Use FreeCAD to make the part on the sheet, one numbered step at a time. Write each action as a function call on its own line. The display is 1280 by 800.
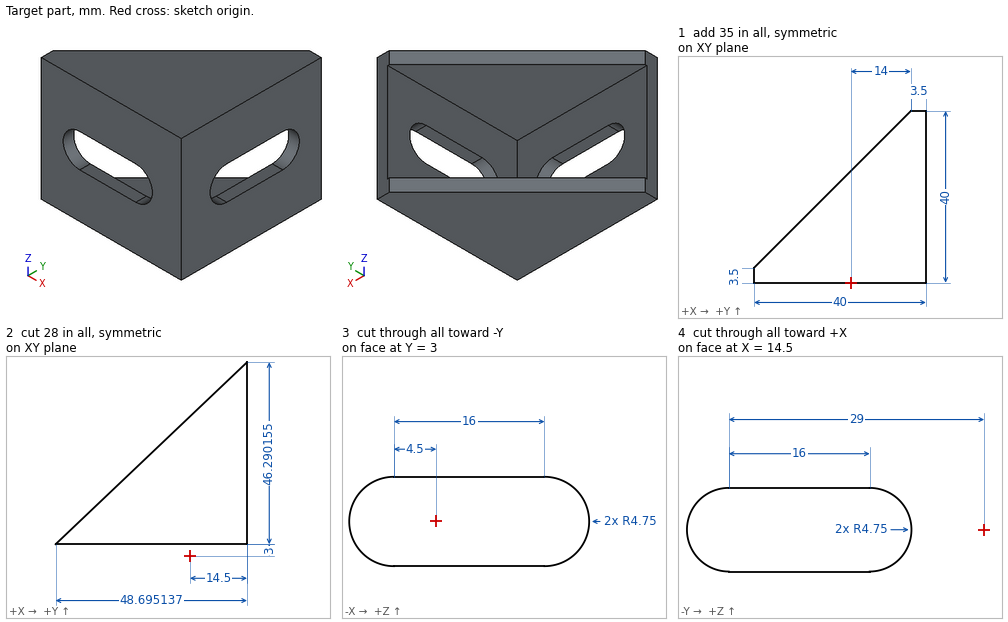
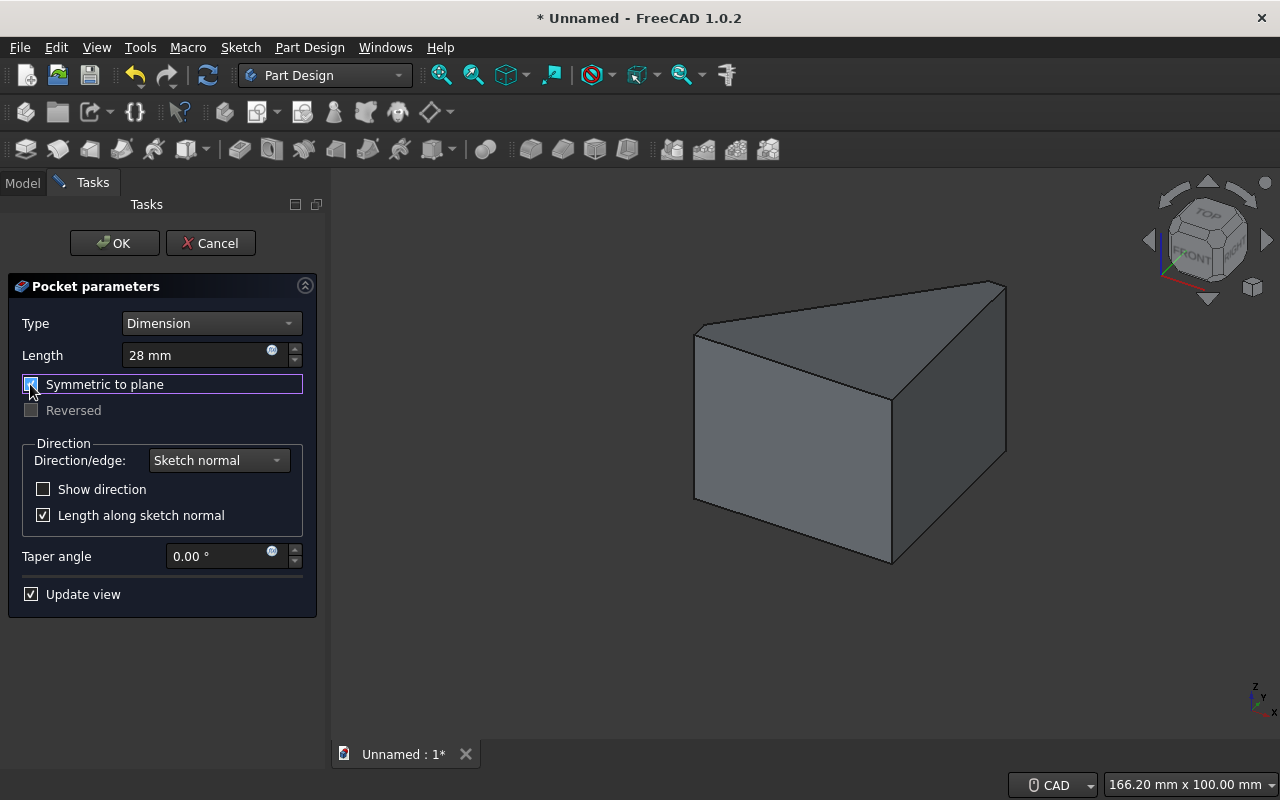
click(115, 243)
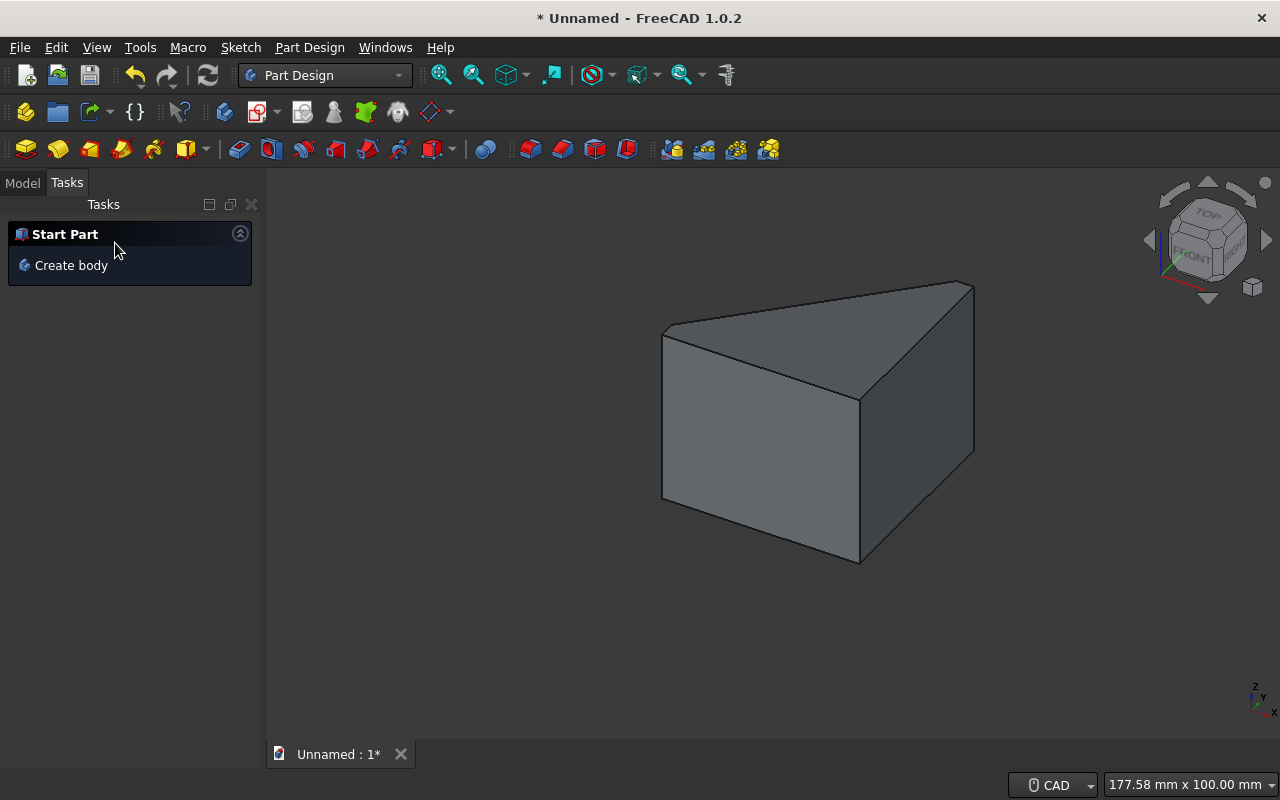
key(4)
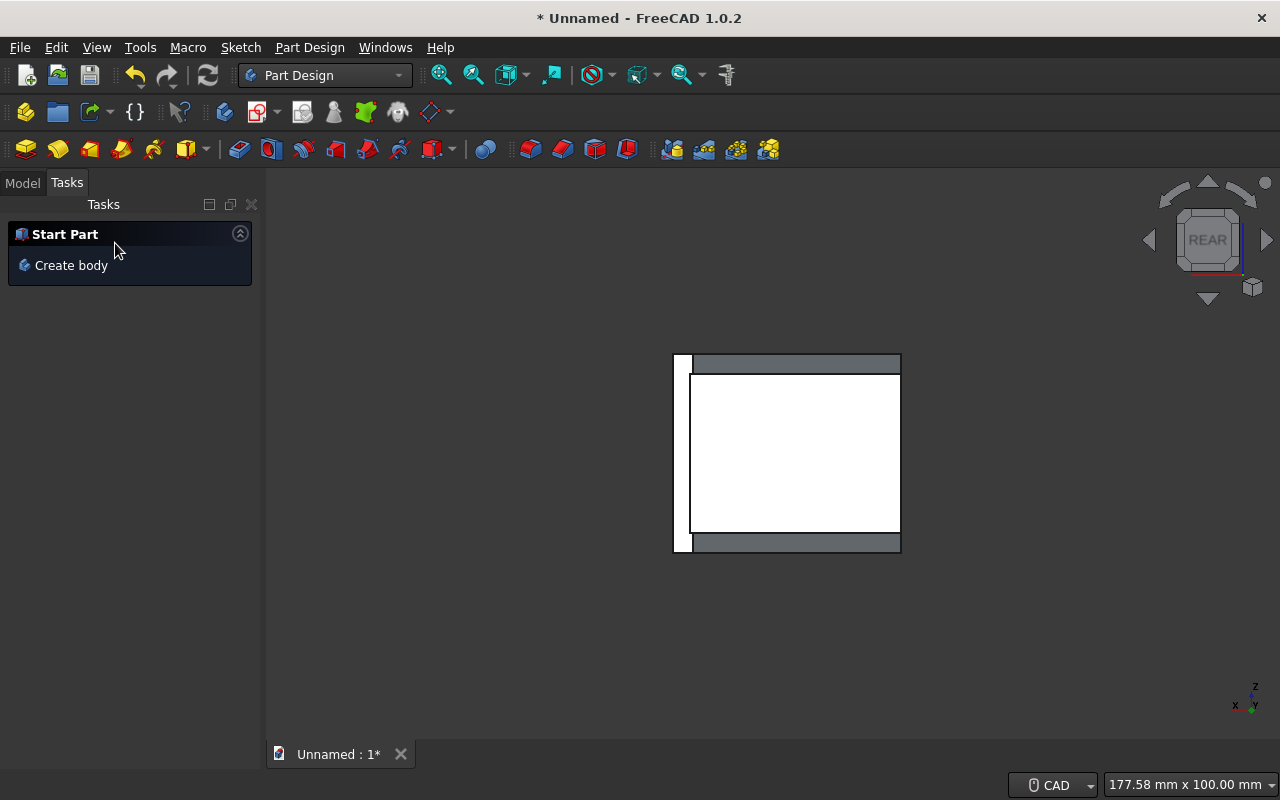
click(442, 76)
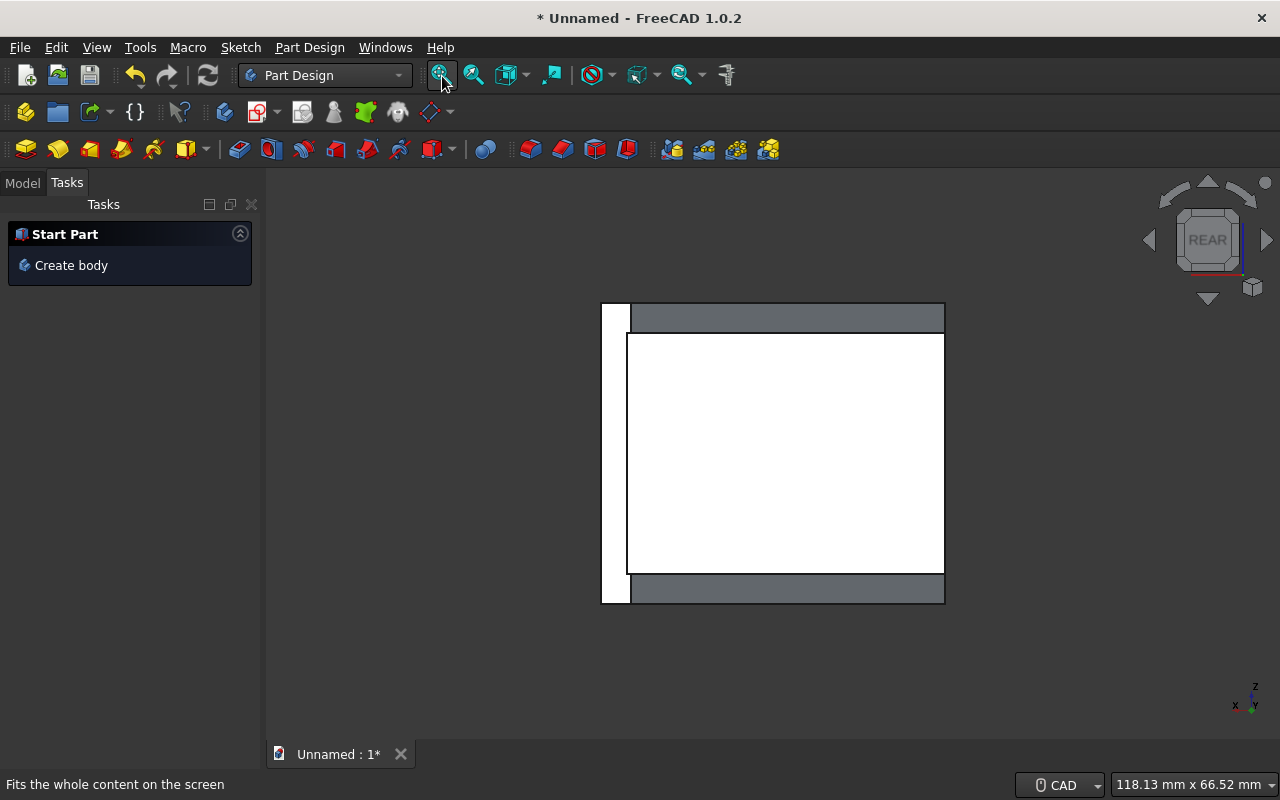
click(786, 453)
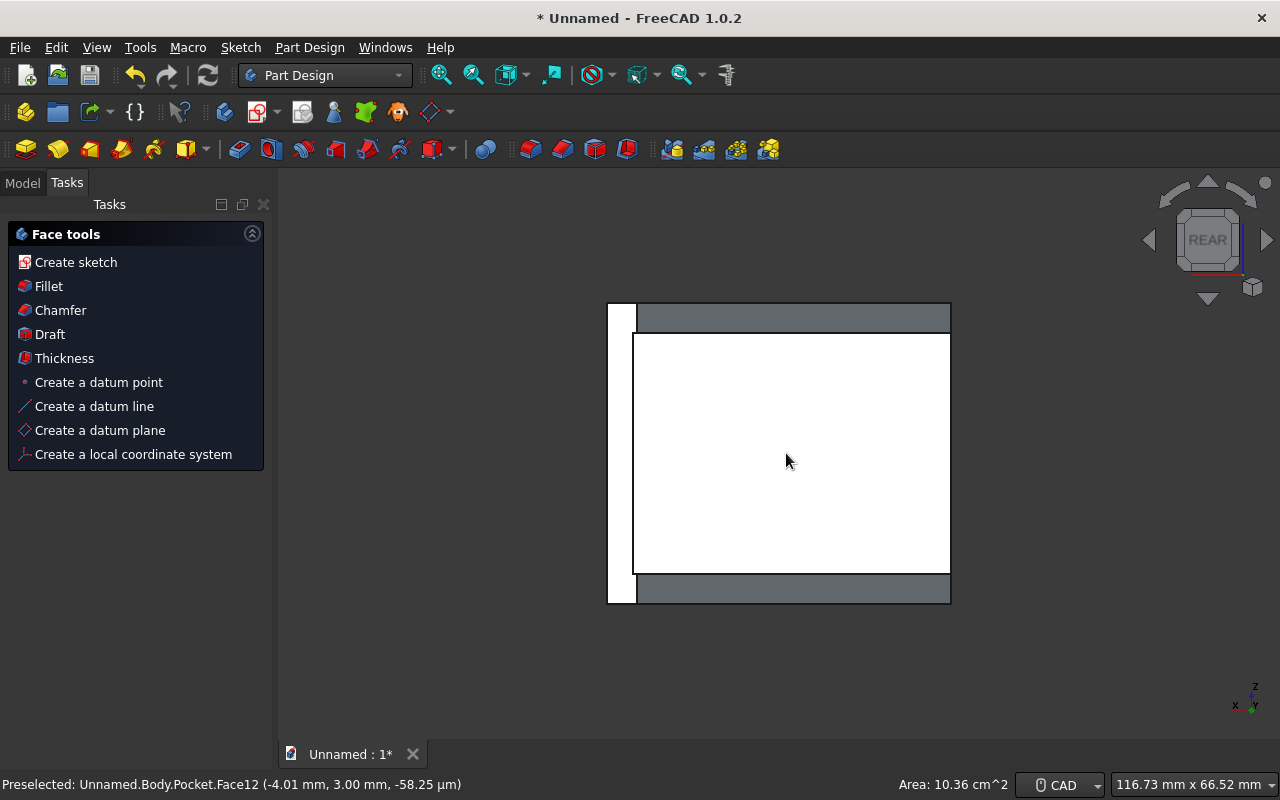
click(258, 112)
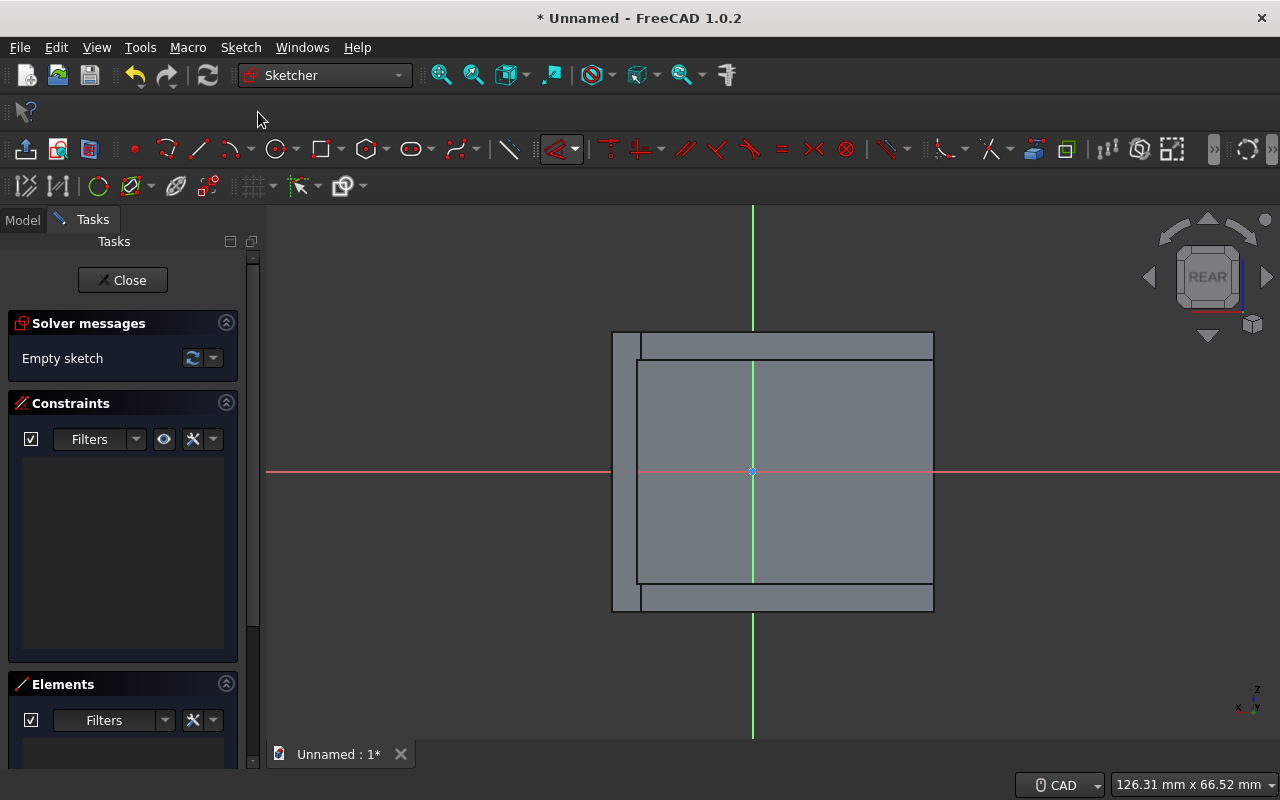
scroll(826, 472, up, 5)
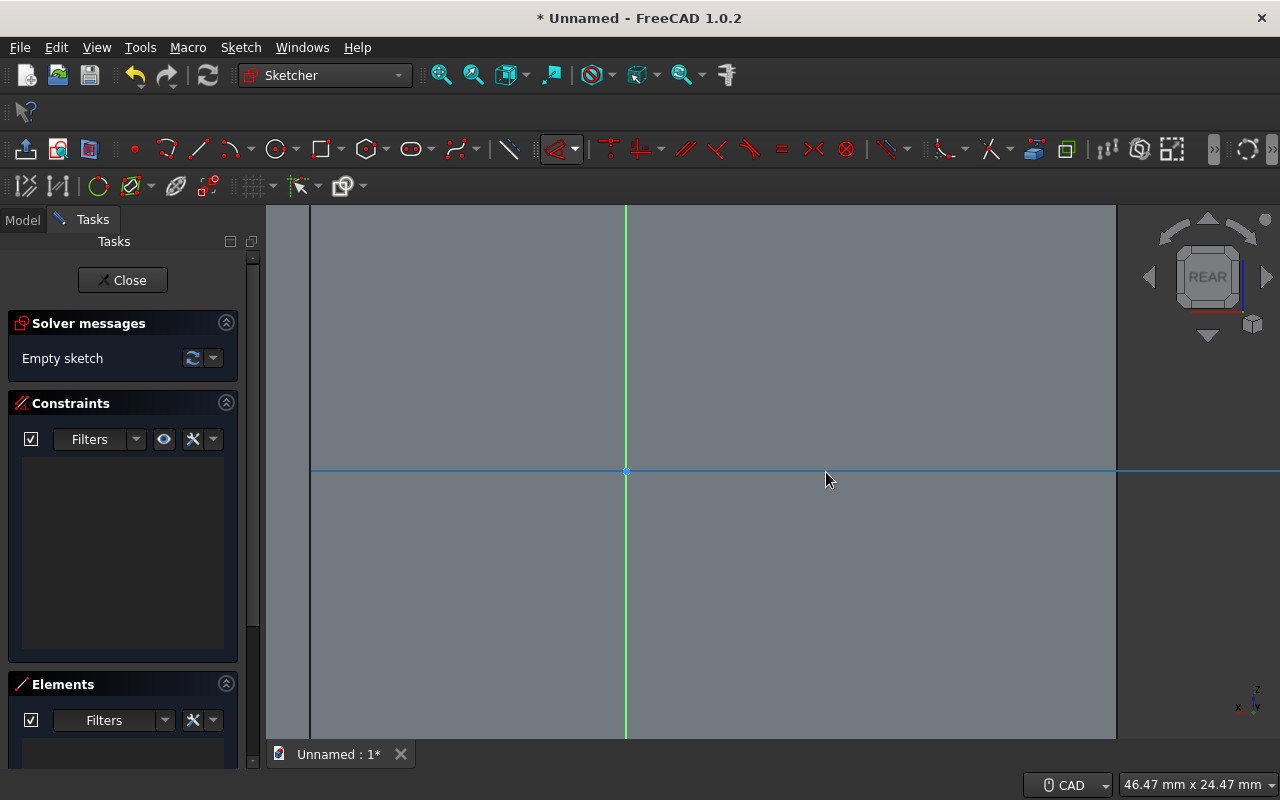
click(412, 150)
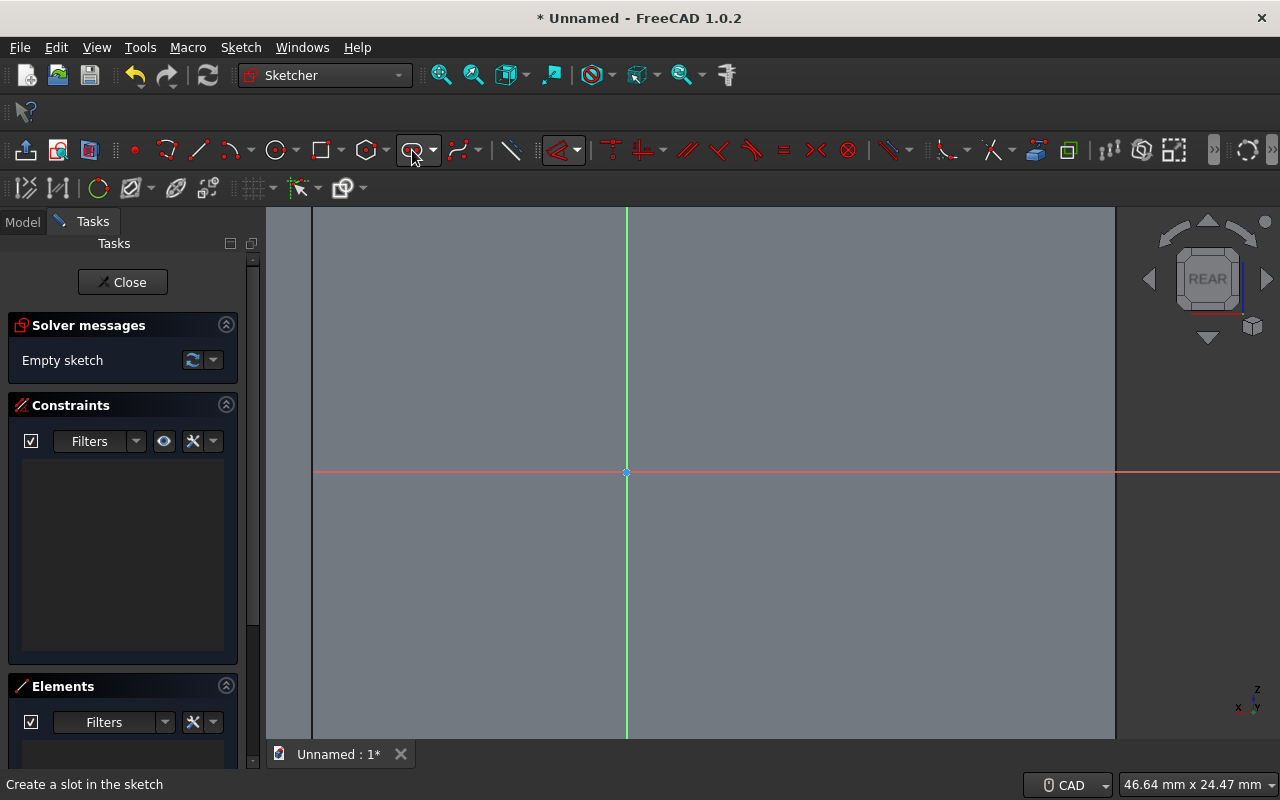
click(529, 472)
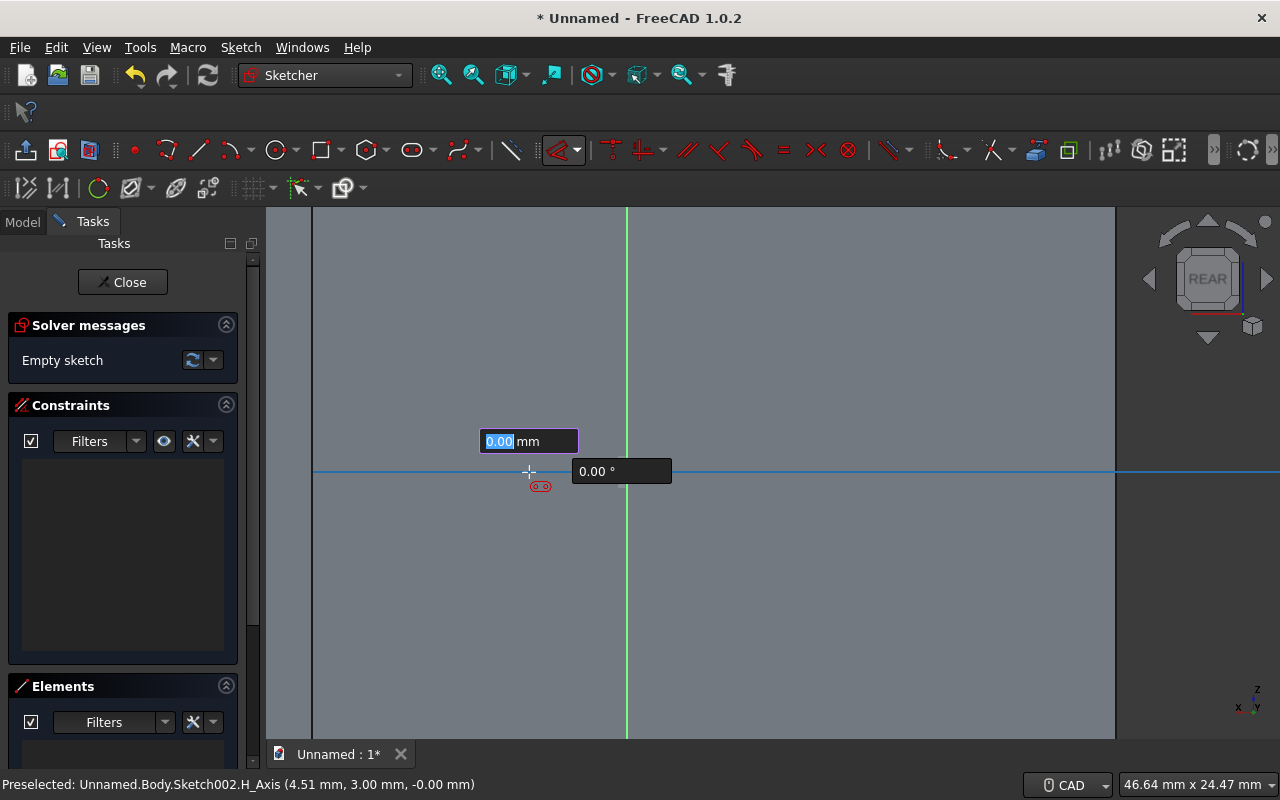
click(877, 463)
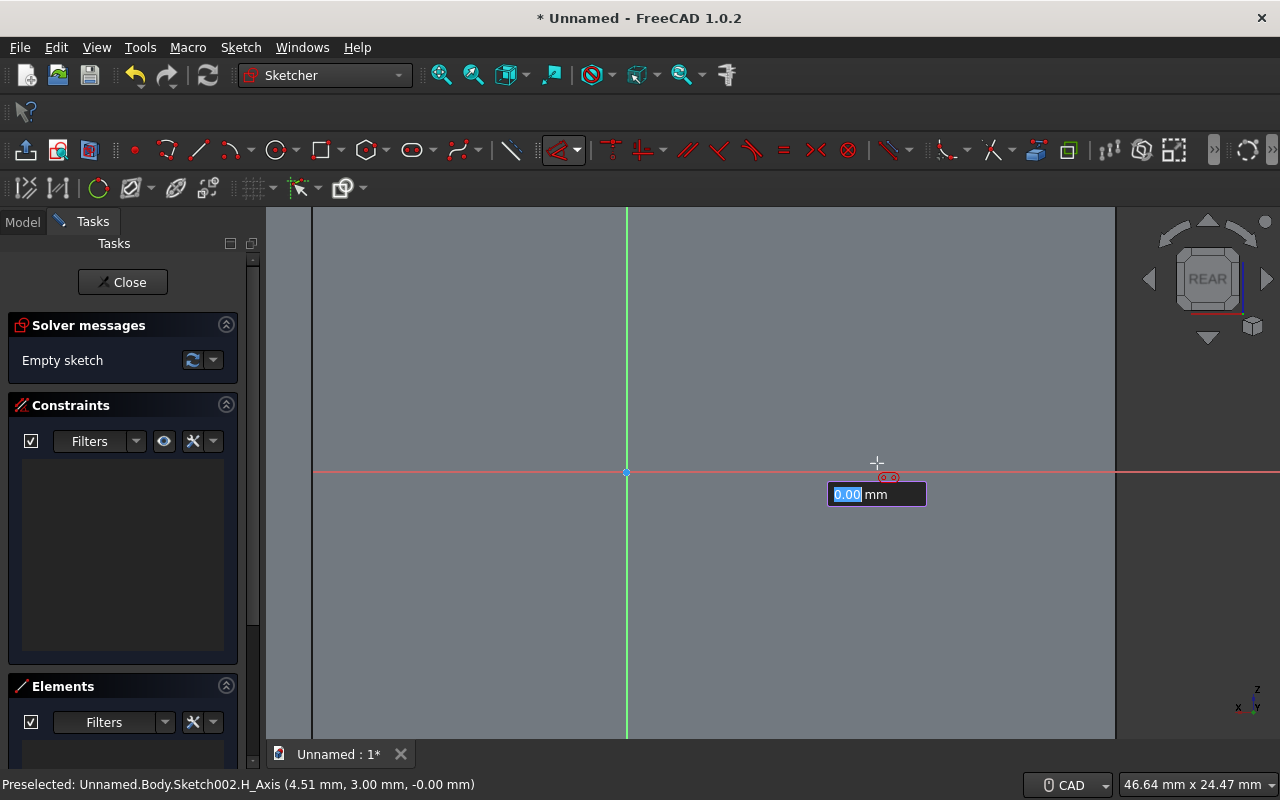
click(703, 575)
key(Escape)